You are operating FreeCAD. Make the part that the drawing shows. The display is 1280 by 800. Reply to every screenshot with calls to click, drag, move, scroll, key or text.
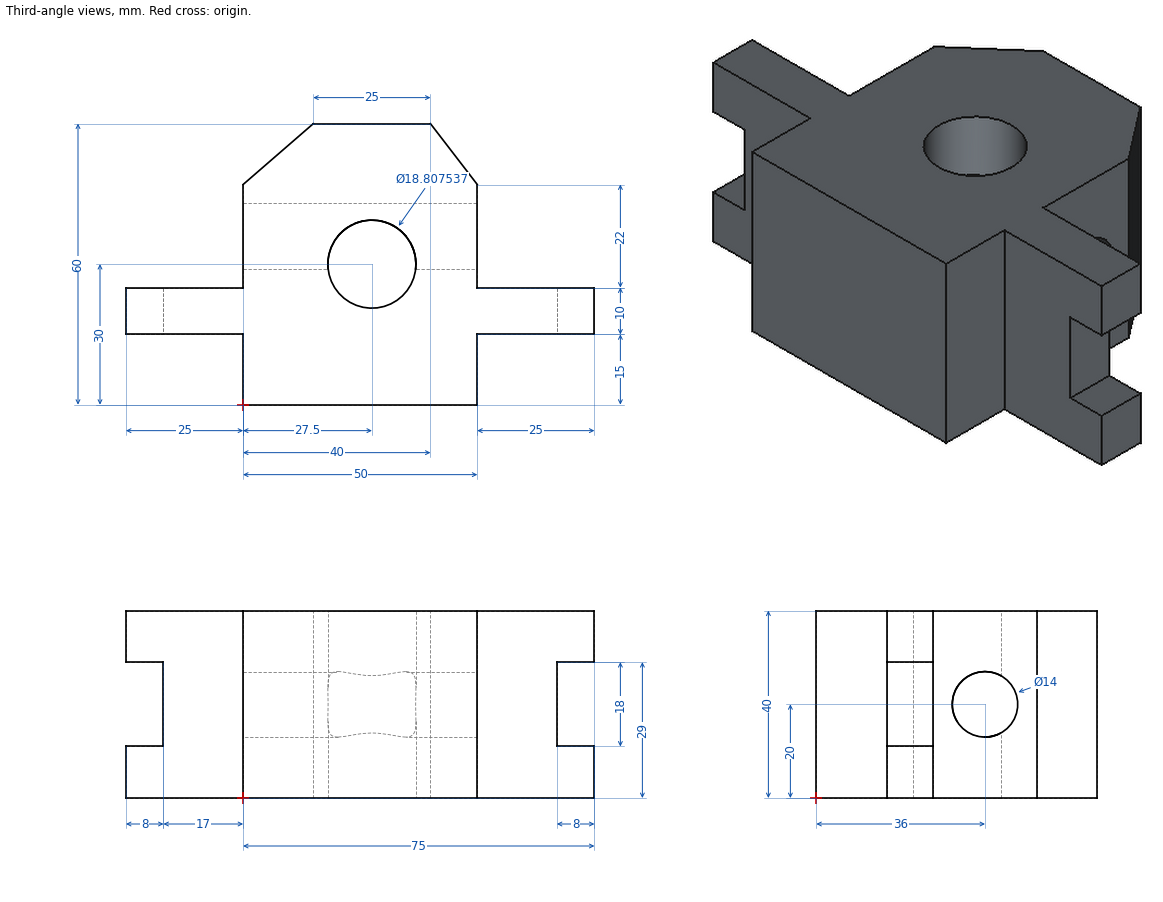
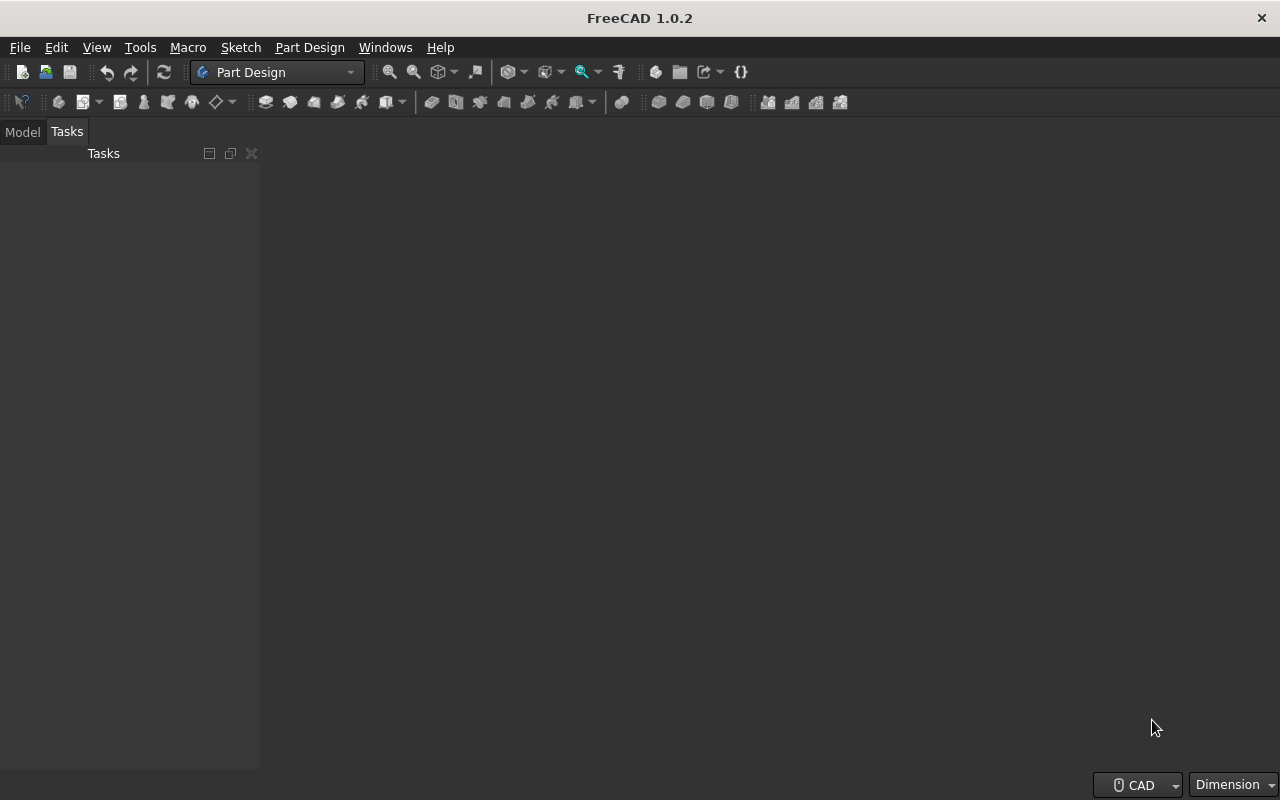
click(22, 72)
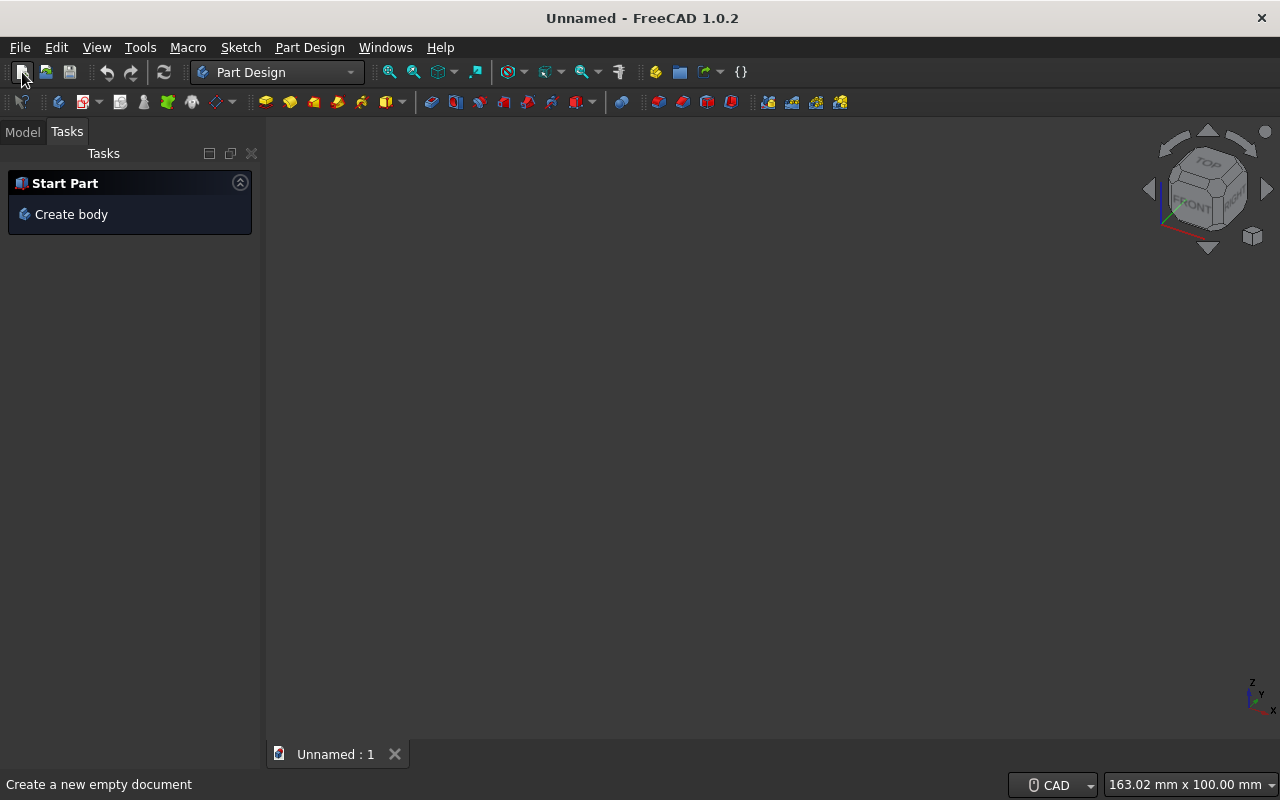
click(84, 102)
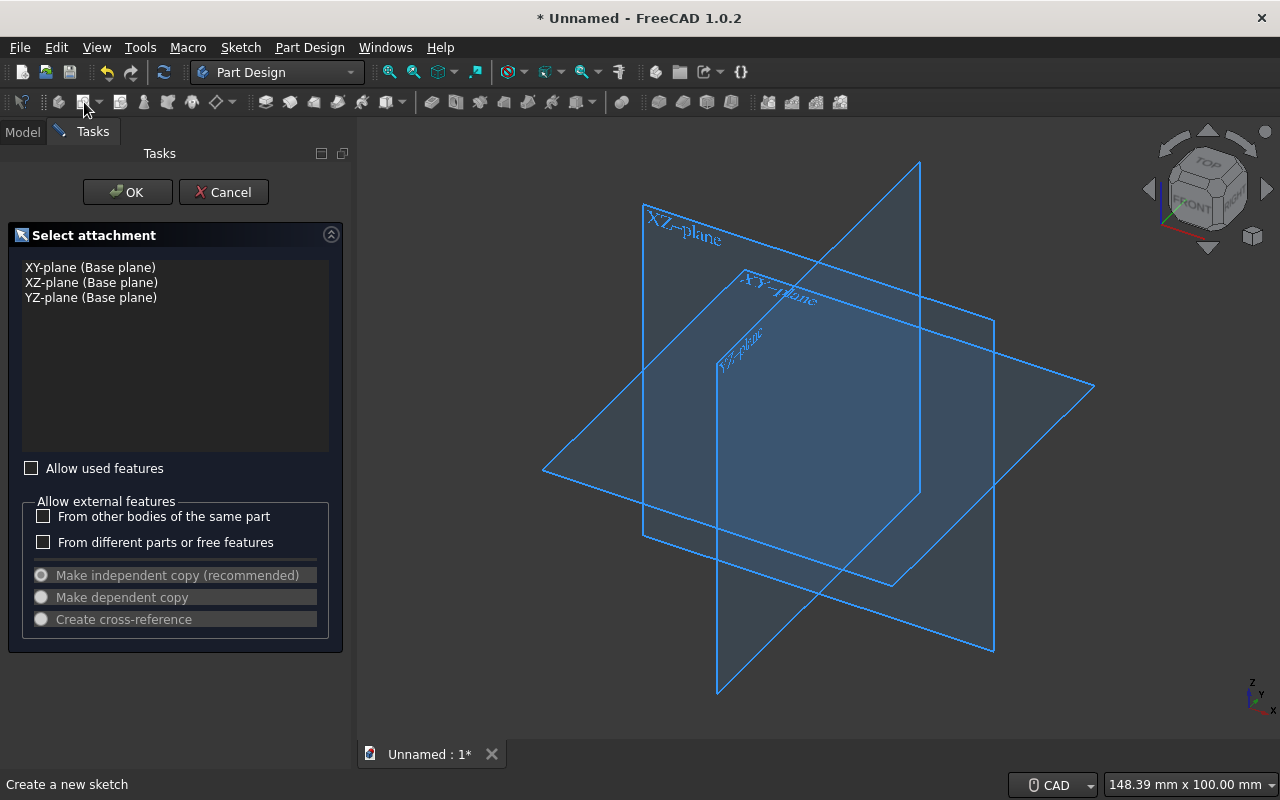
click(82, 268)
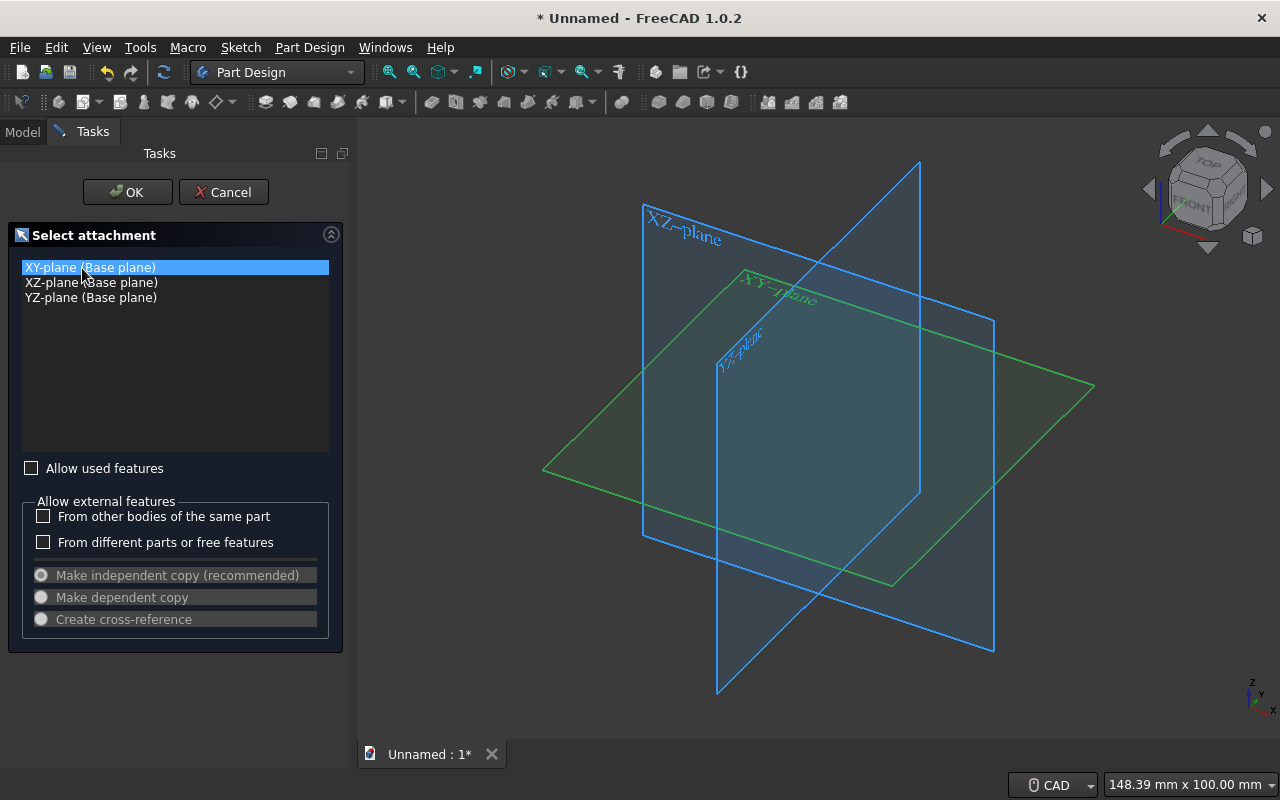
click(128, 192)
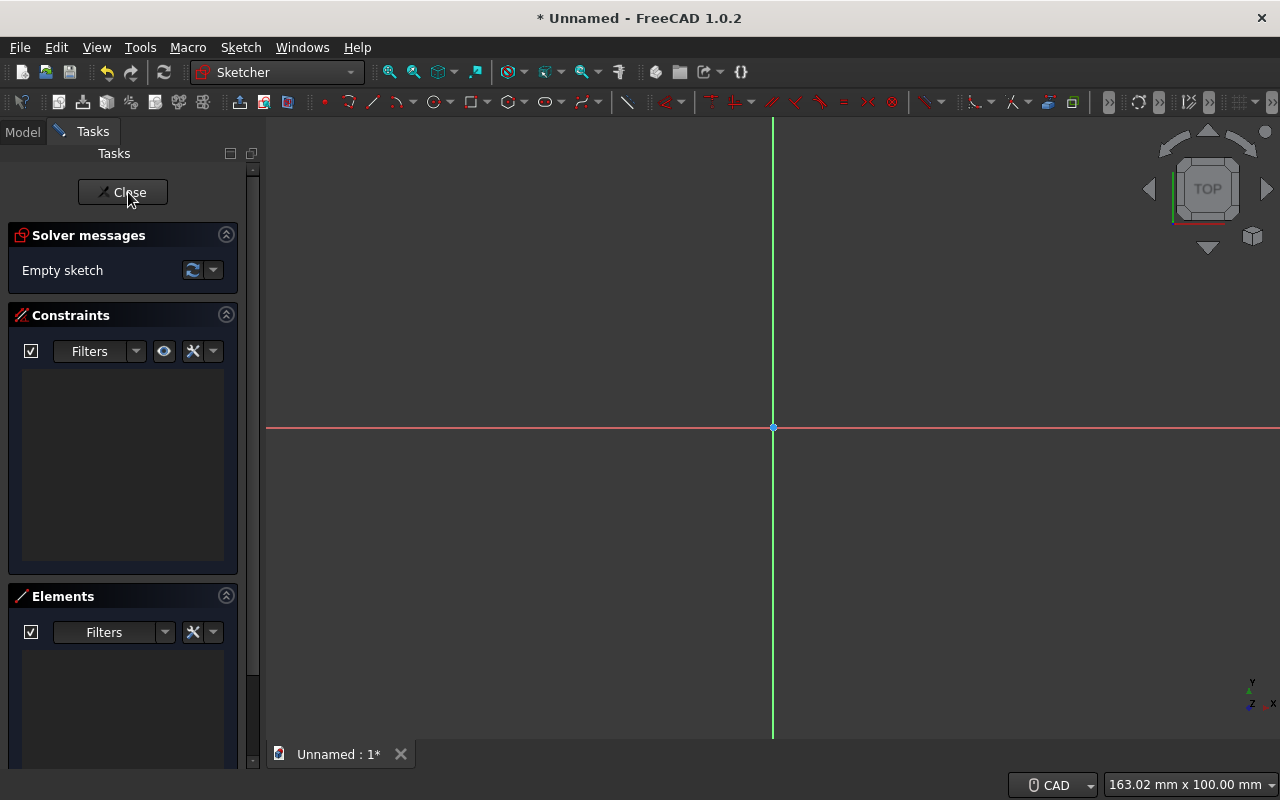
scroll(294, 711, down, 1)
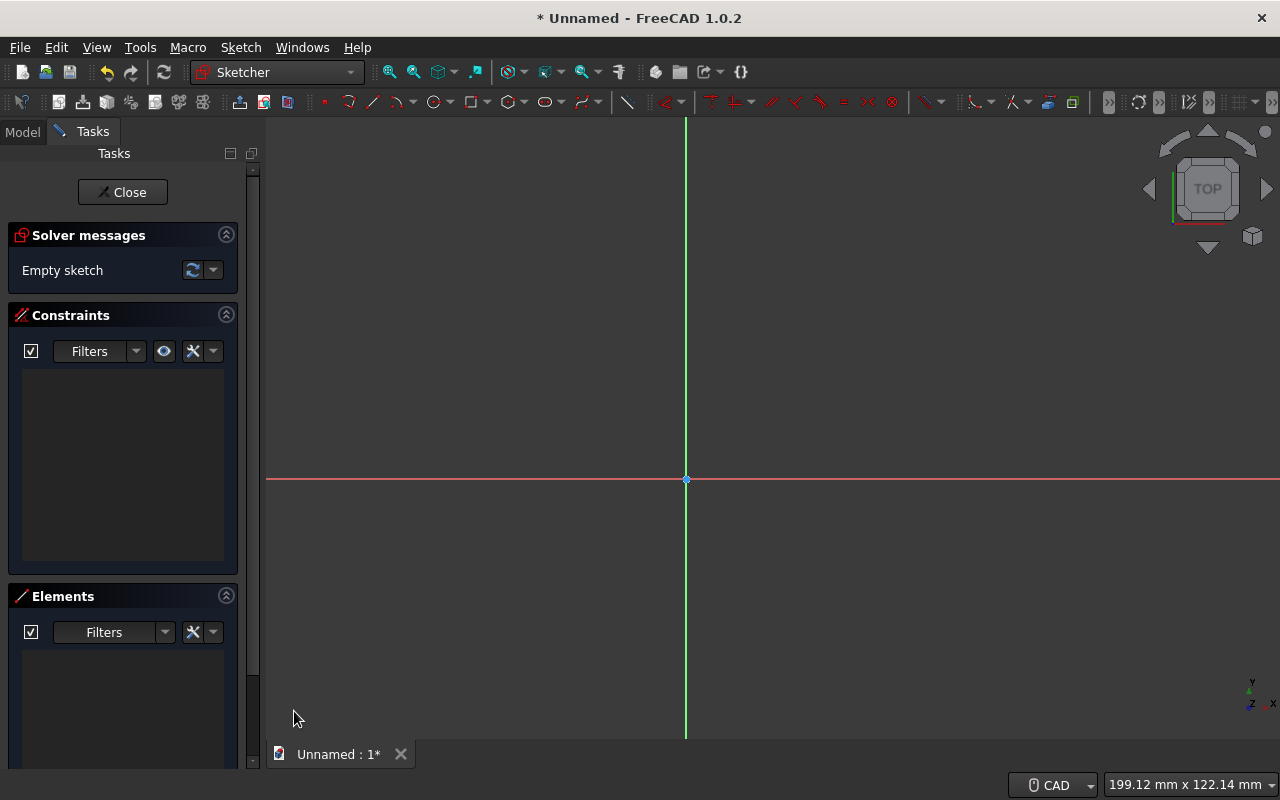
key(g)
key(m)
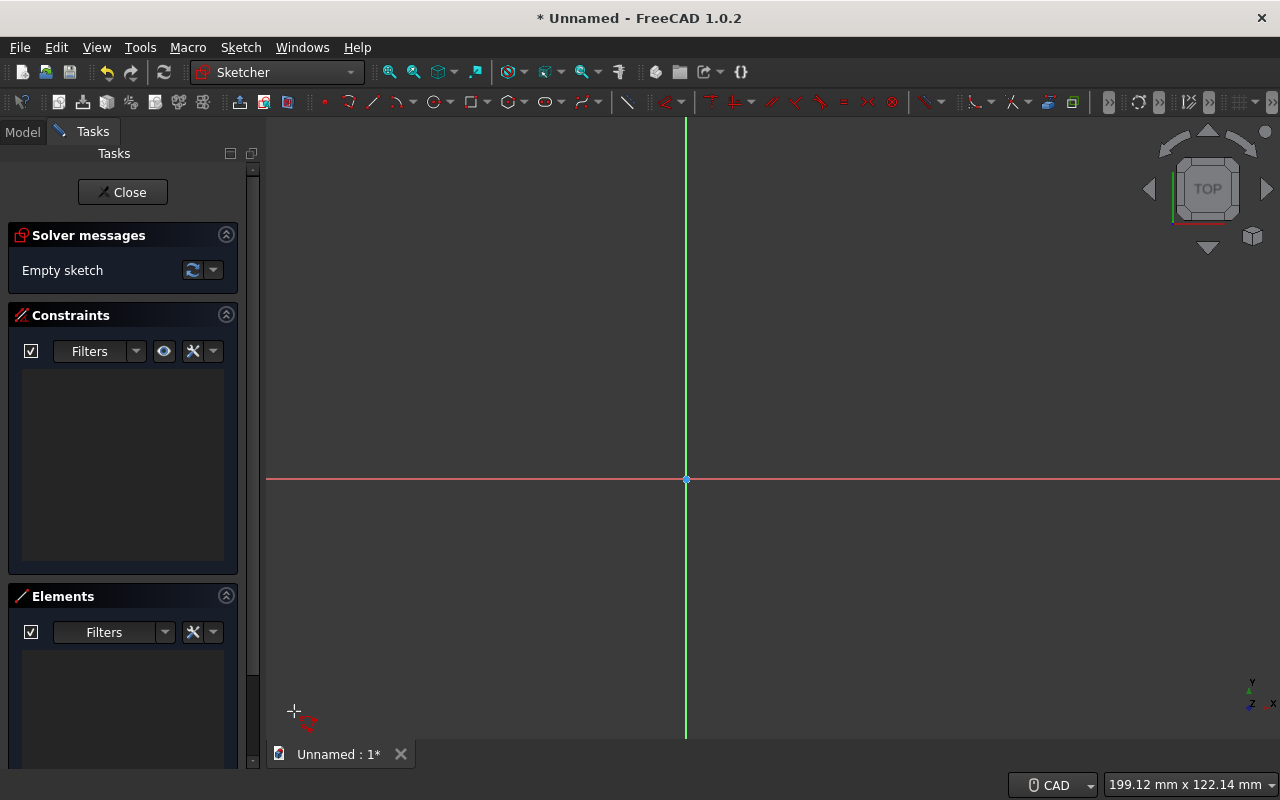
click(686, 479)
click(941, 470)
click(941, 403)
click(1068, 403)
click(1068, 352)
click(941, 352)
click(941, 240)
click(890, 174)
click(763, 174)
click(686, 240)
click(695, 352)
click(559, 352)
click(559, 403)
click(695, 403)
click(686, 479)
key(Escape)
key(Escape)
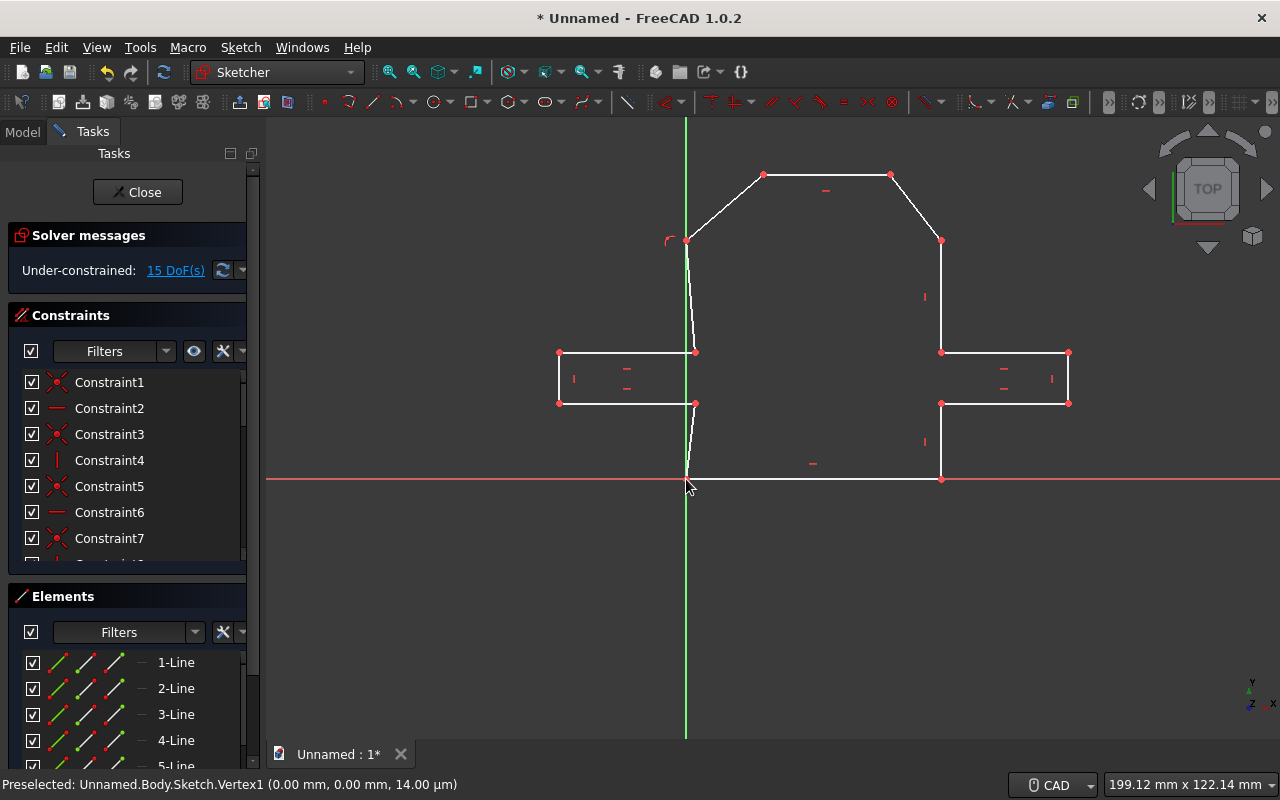
click(689, 275)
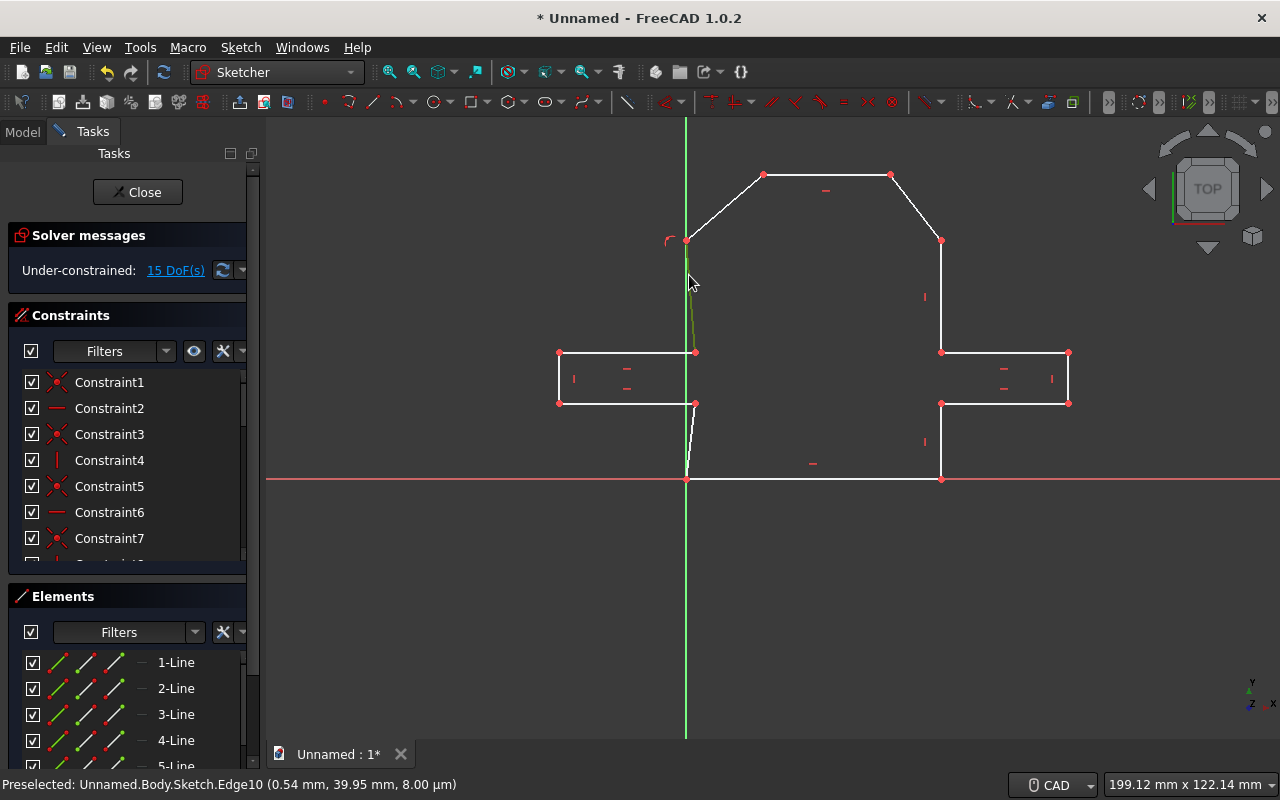
key(v)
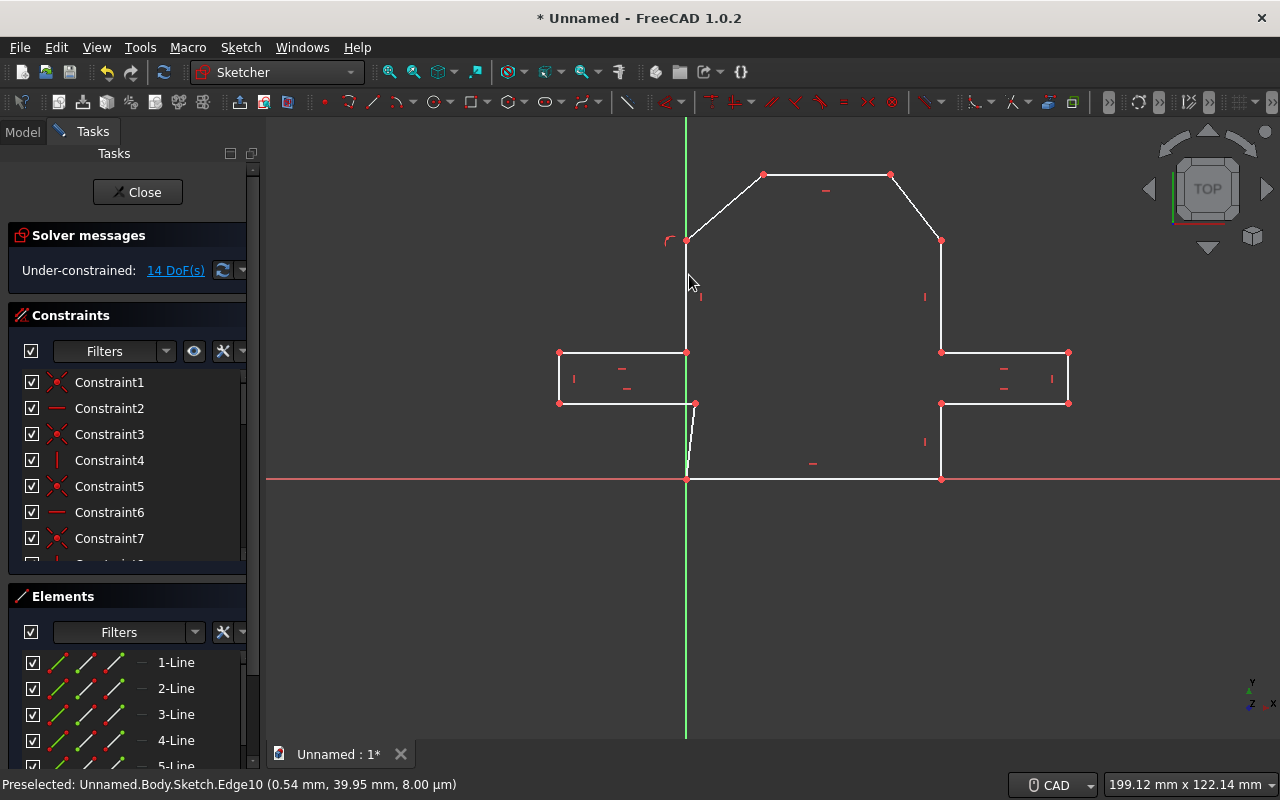
click(689, 457)